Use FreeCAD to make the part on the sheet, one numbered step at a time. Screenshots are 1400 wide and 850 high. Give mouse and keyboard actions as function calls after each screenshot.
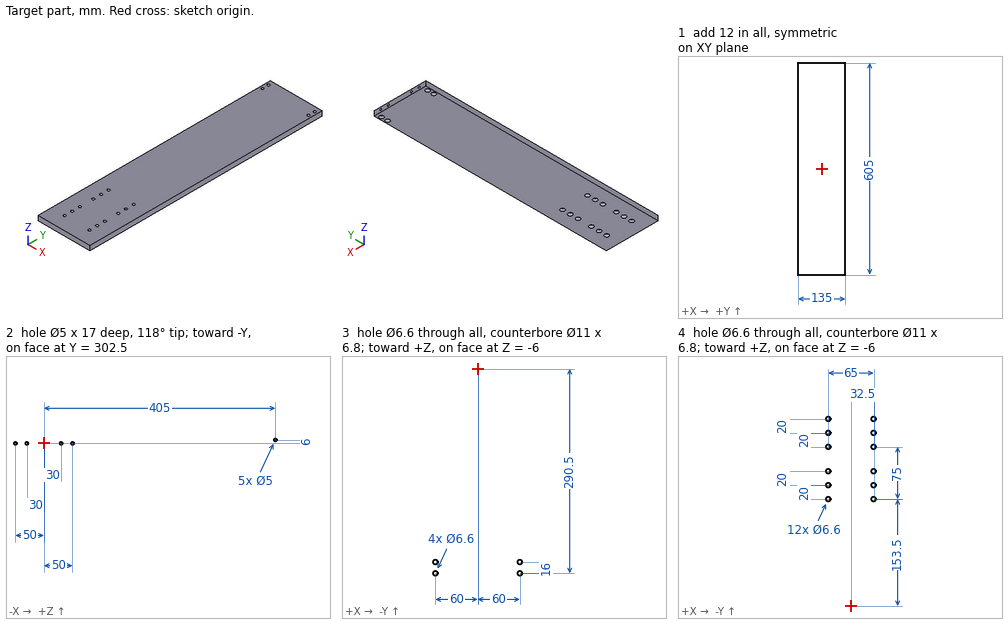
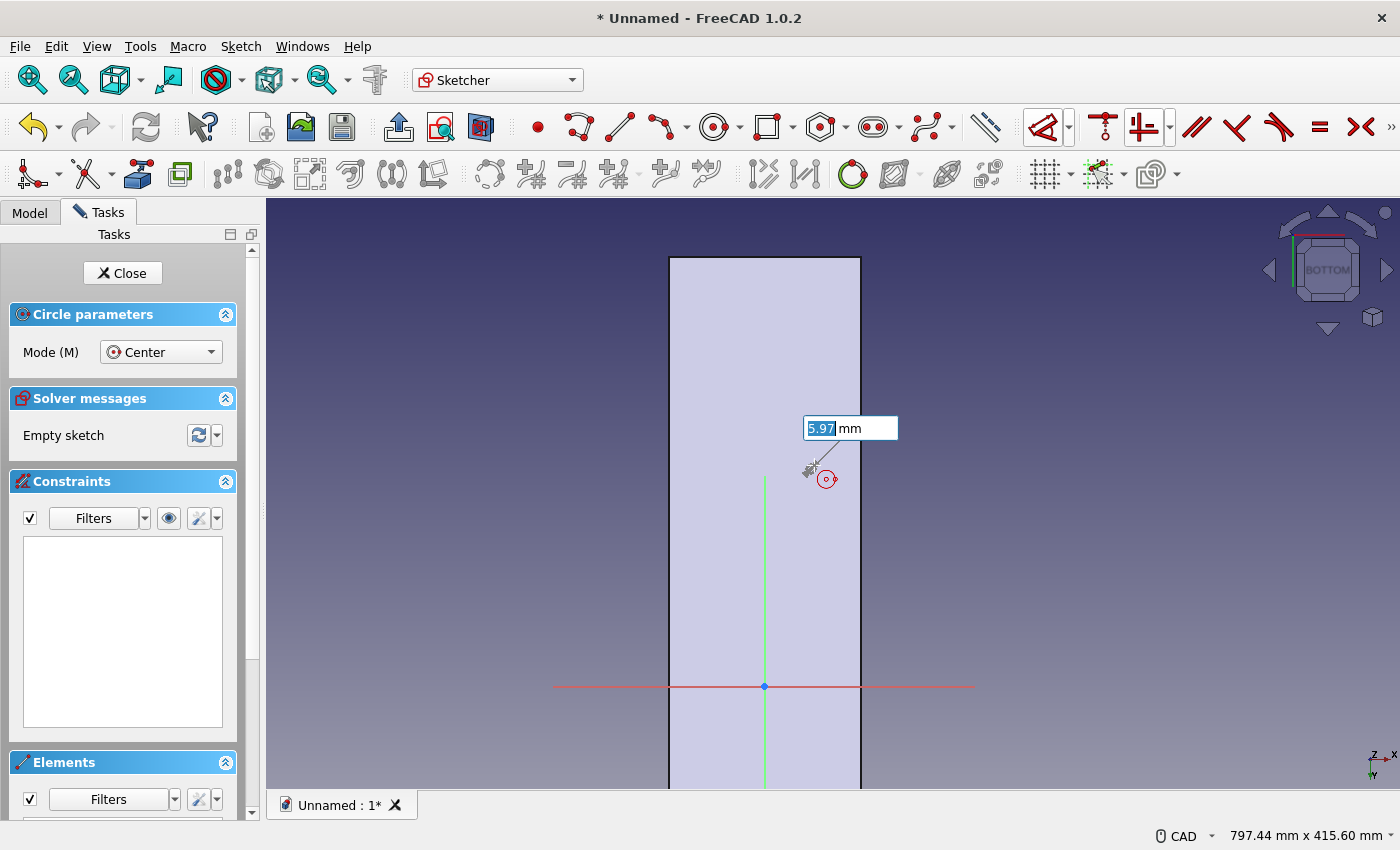
text(6.6)
key(Return)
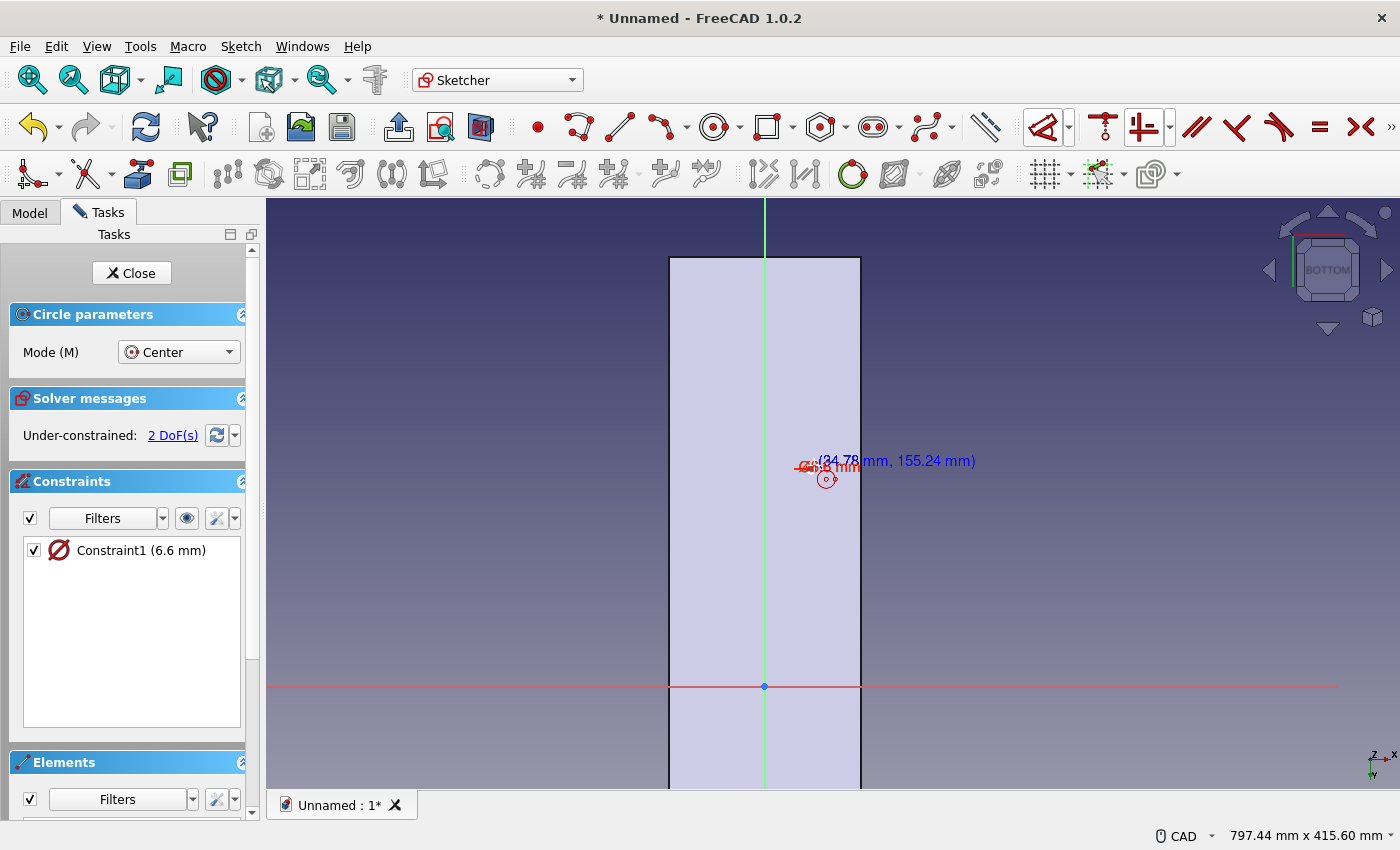
scroll(811, 362, up, 8)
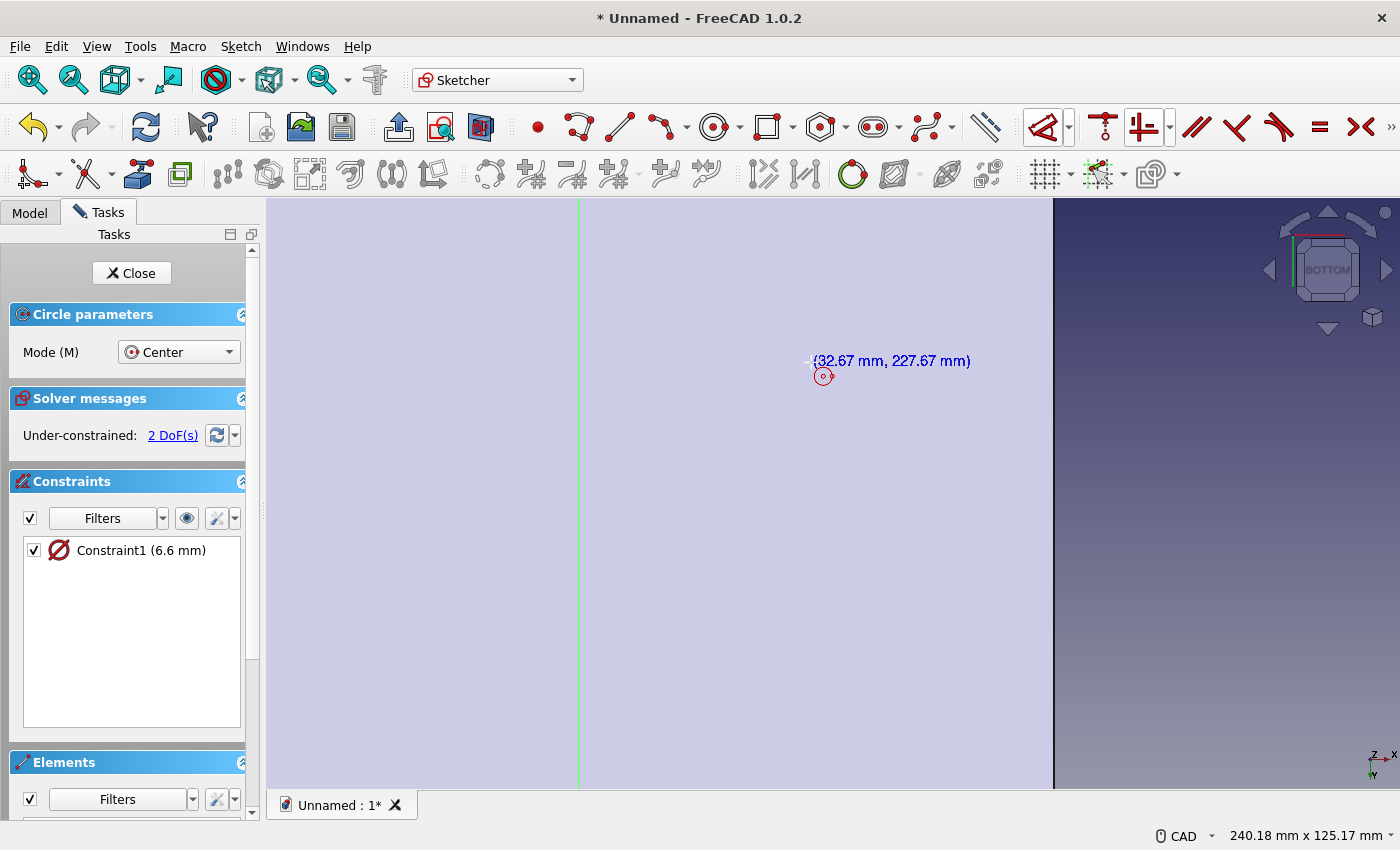
scroll(811, 362, down, 8)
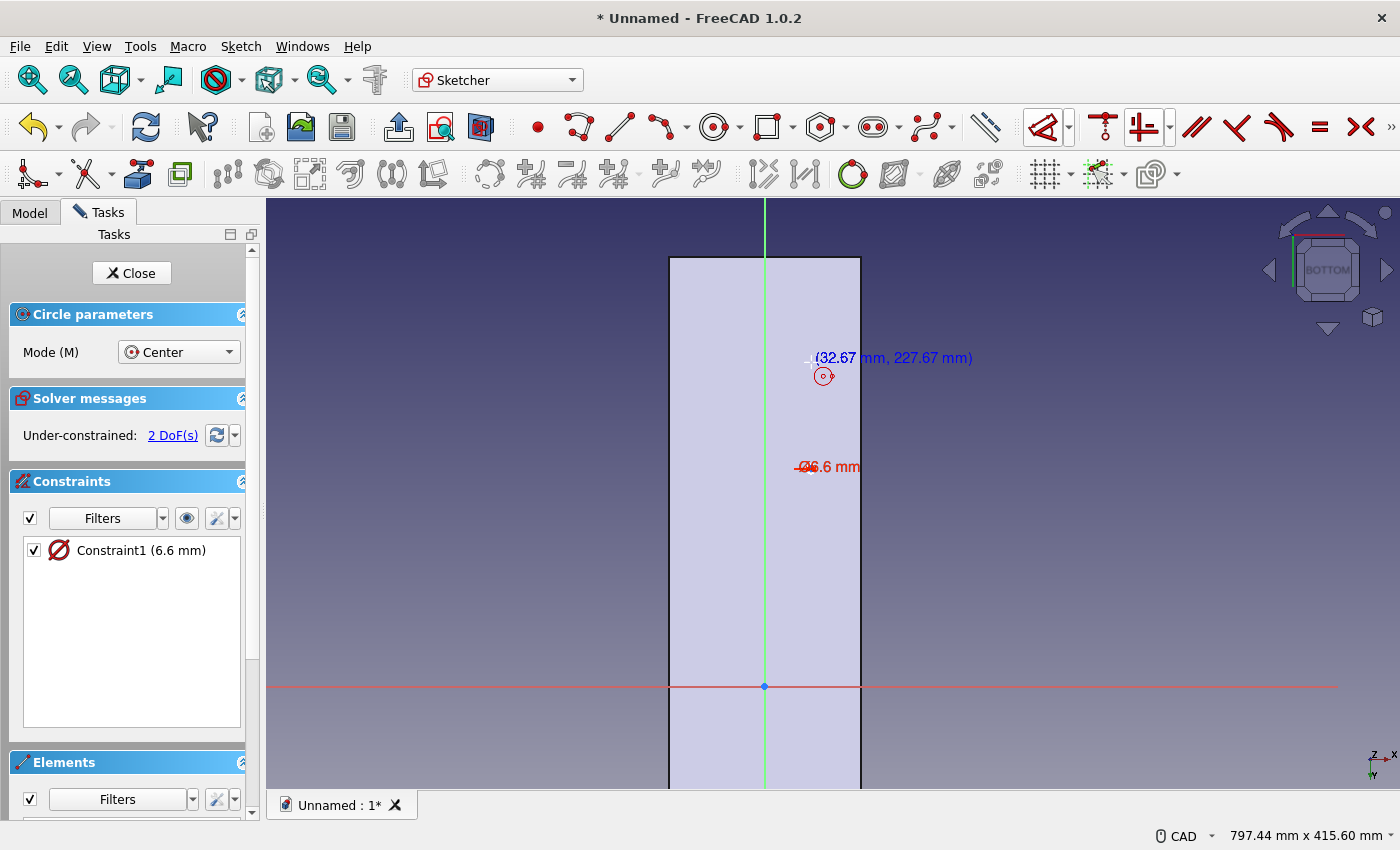
click(811, 362)
move(814, 358)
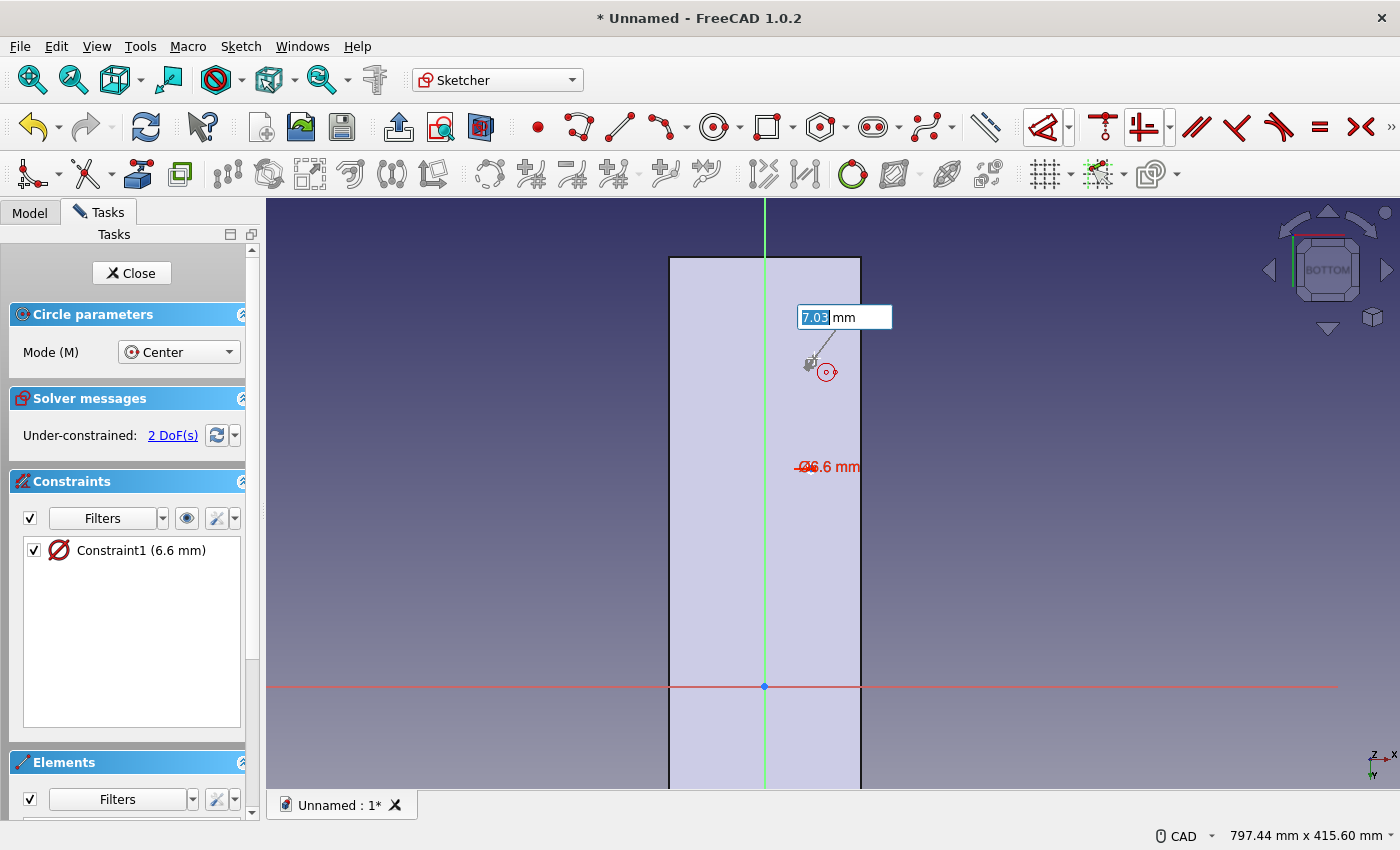
text(6.6)
key(Return)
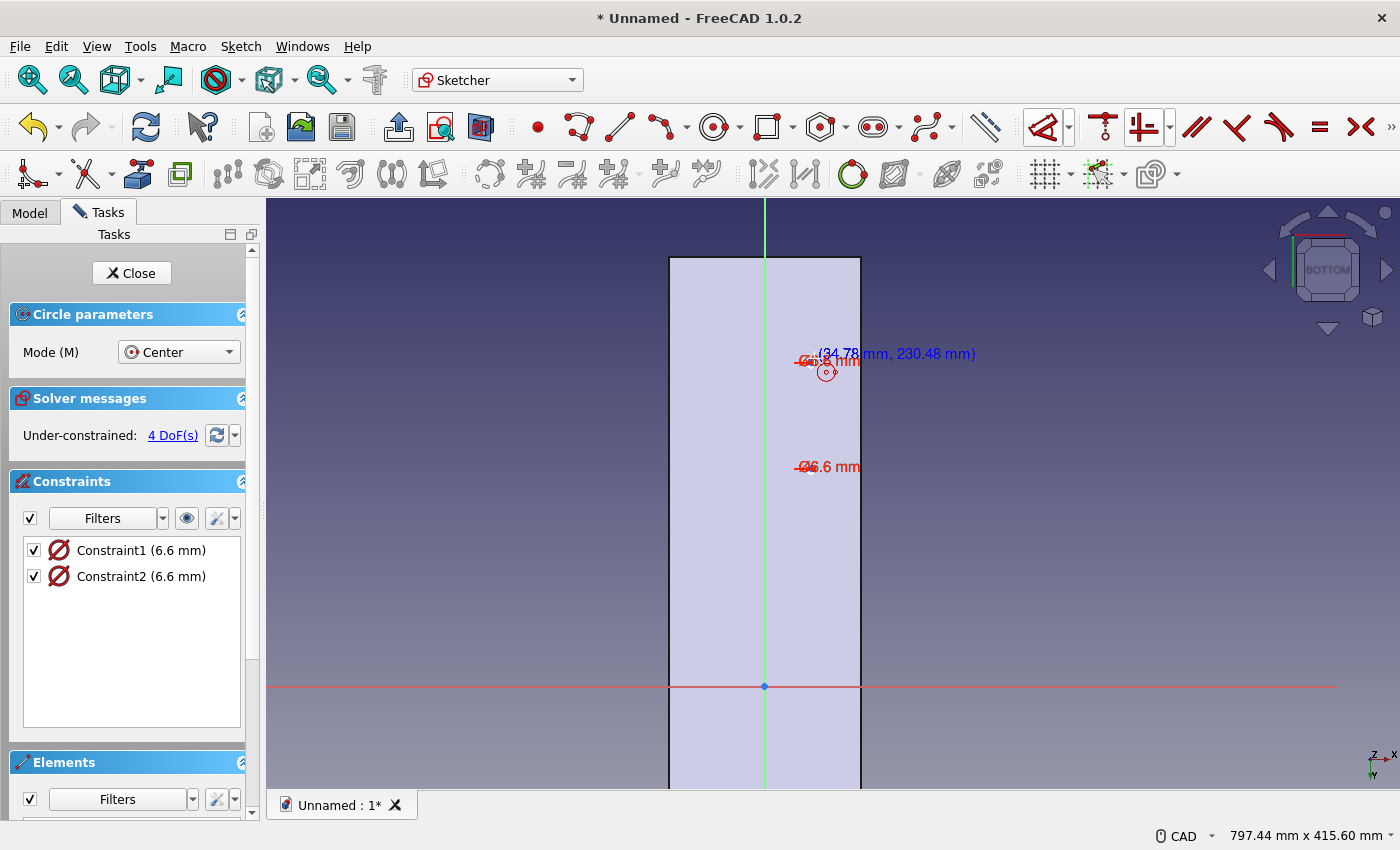
scroll(718, 362, up, 8)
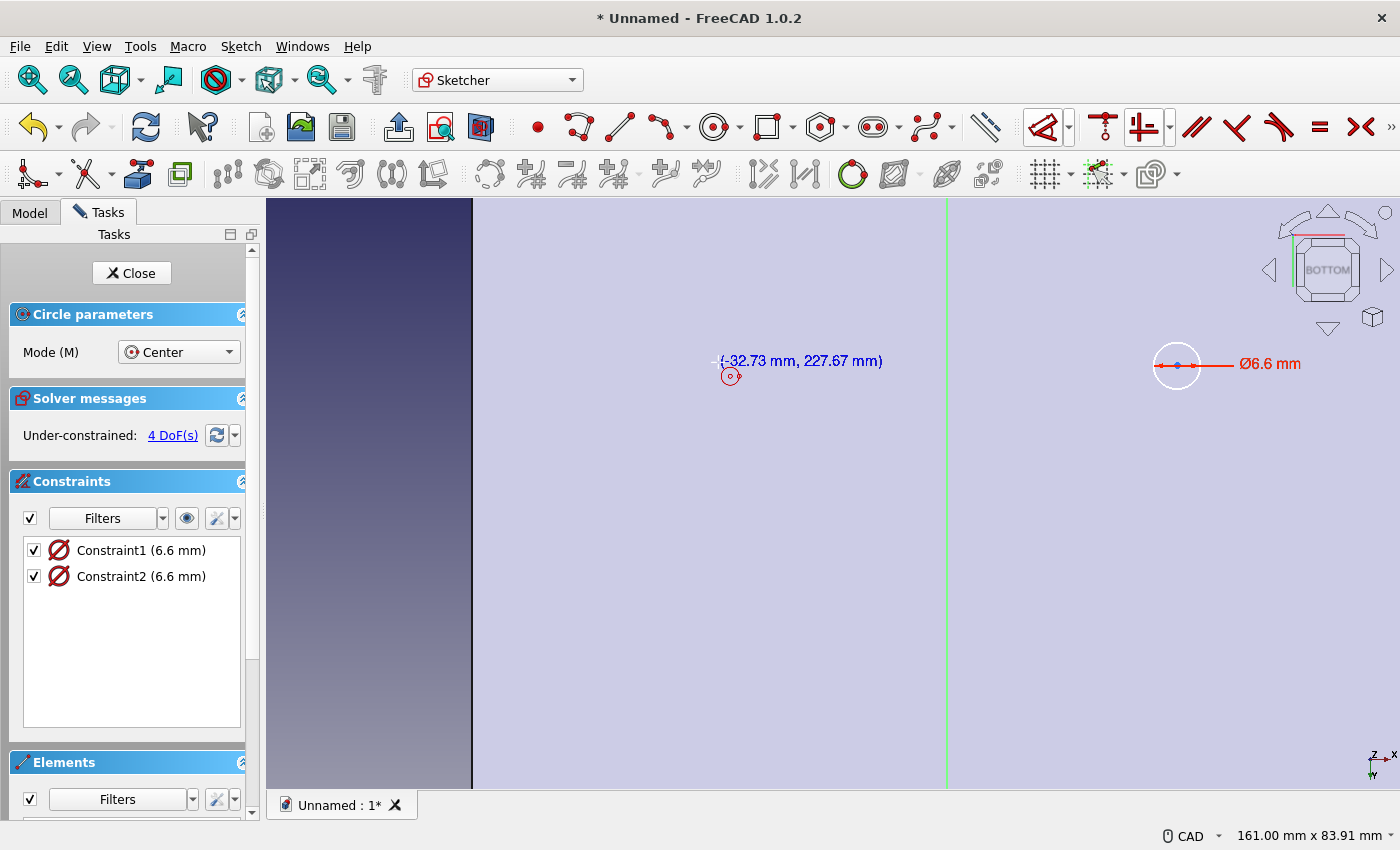
scroll(718, 362, down, 8)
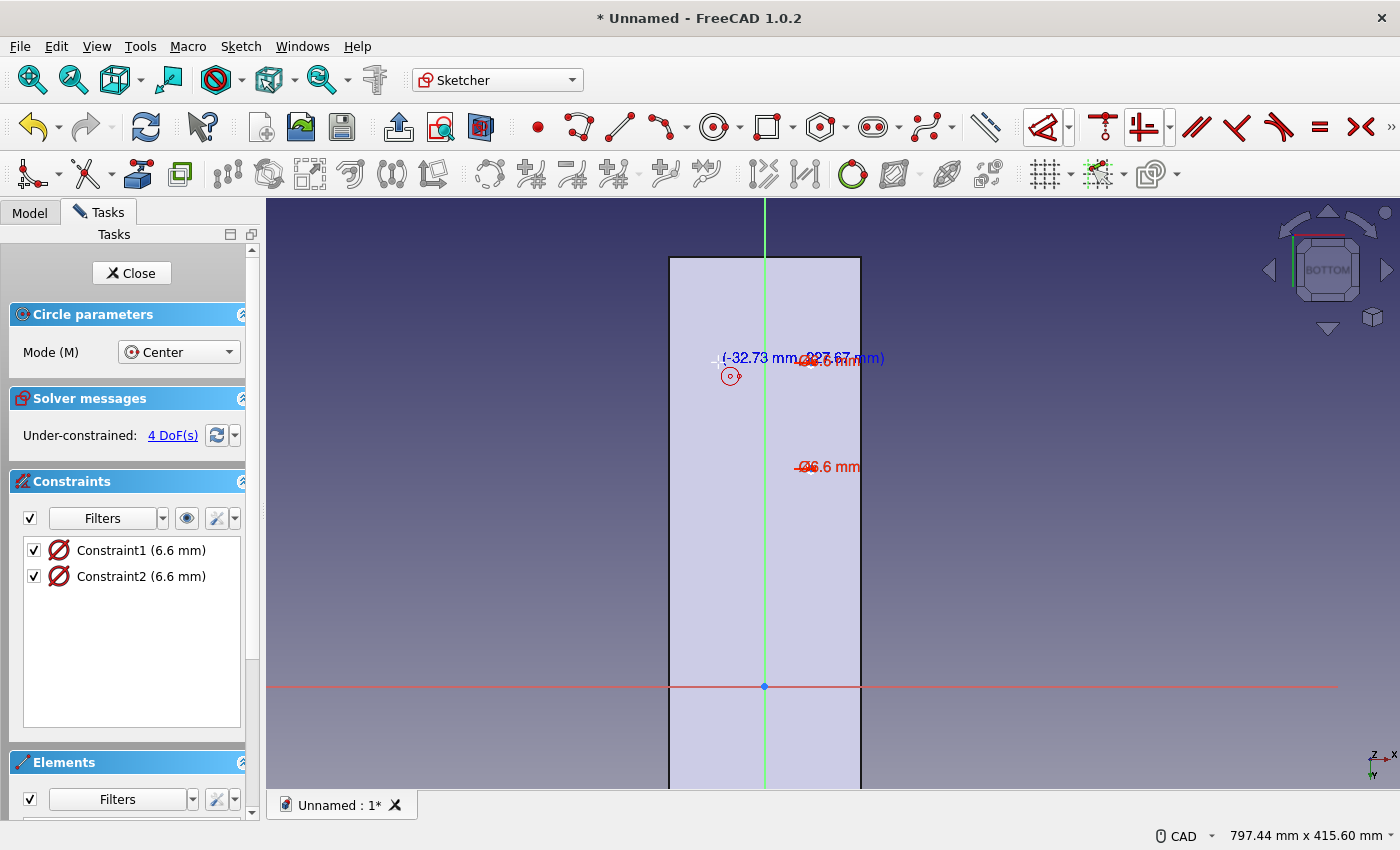
click(718, 362)
move(722, 358)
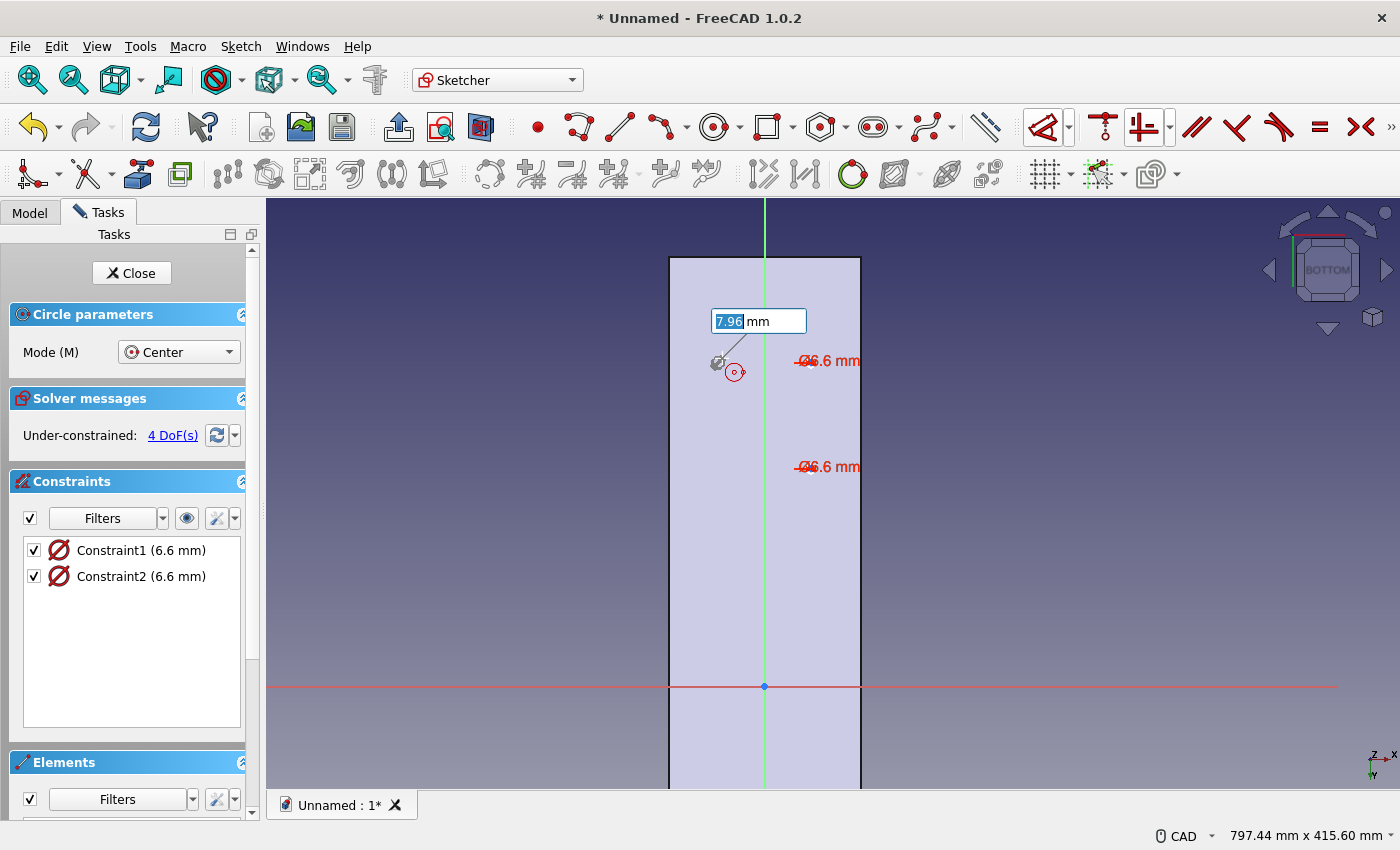
text(6.6)
key(Return)